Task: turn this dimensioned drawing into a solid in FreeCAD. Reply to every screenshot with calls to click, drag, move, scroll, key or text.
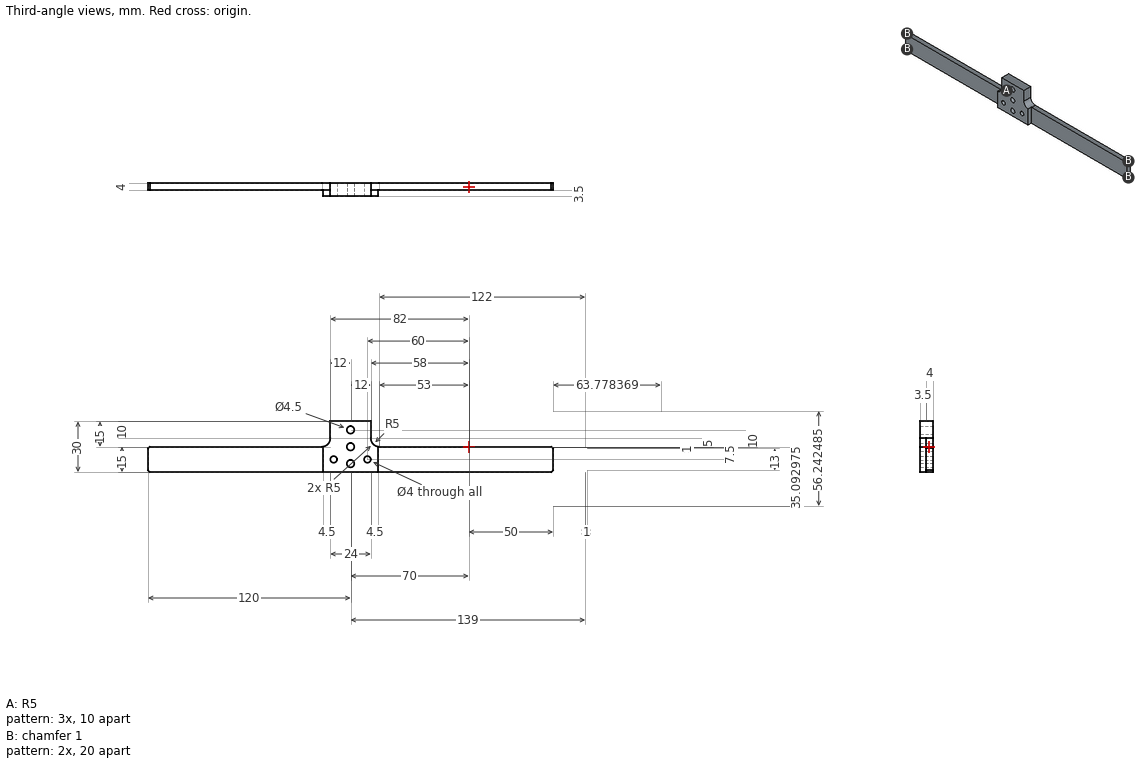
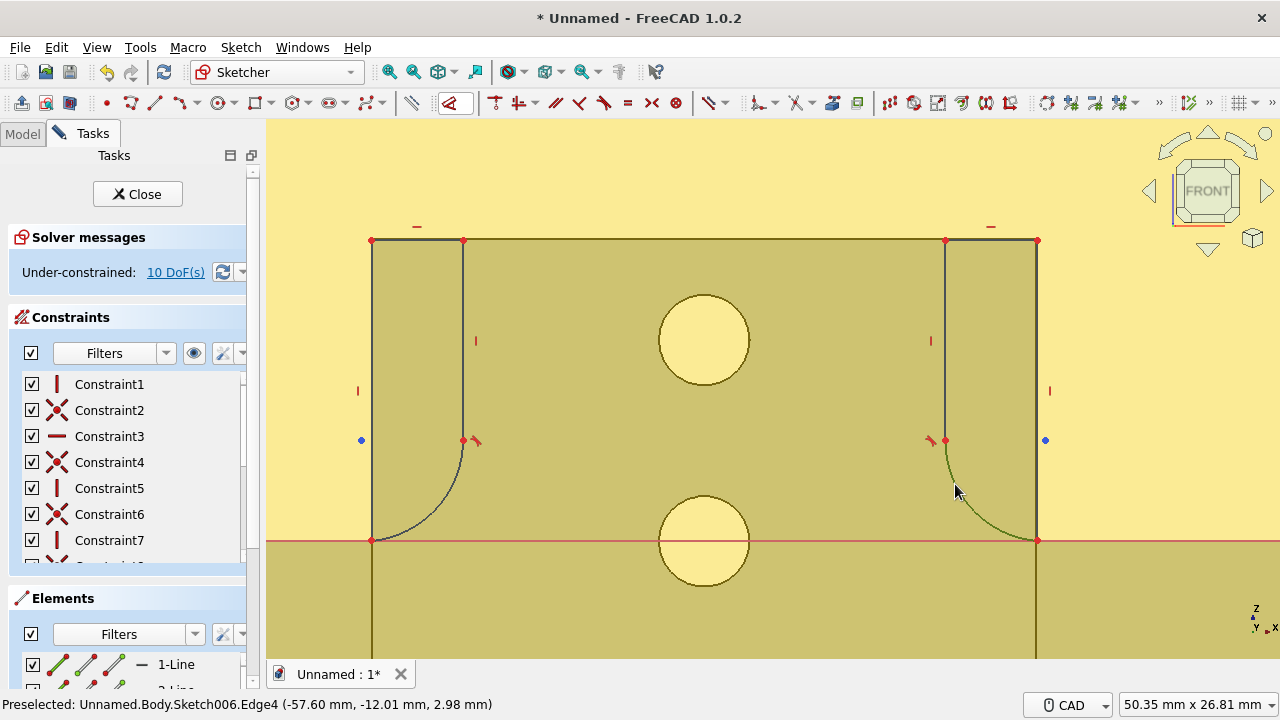
click(414, 527)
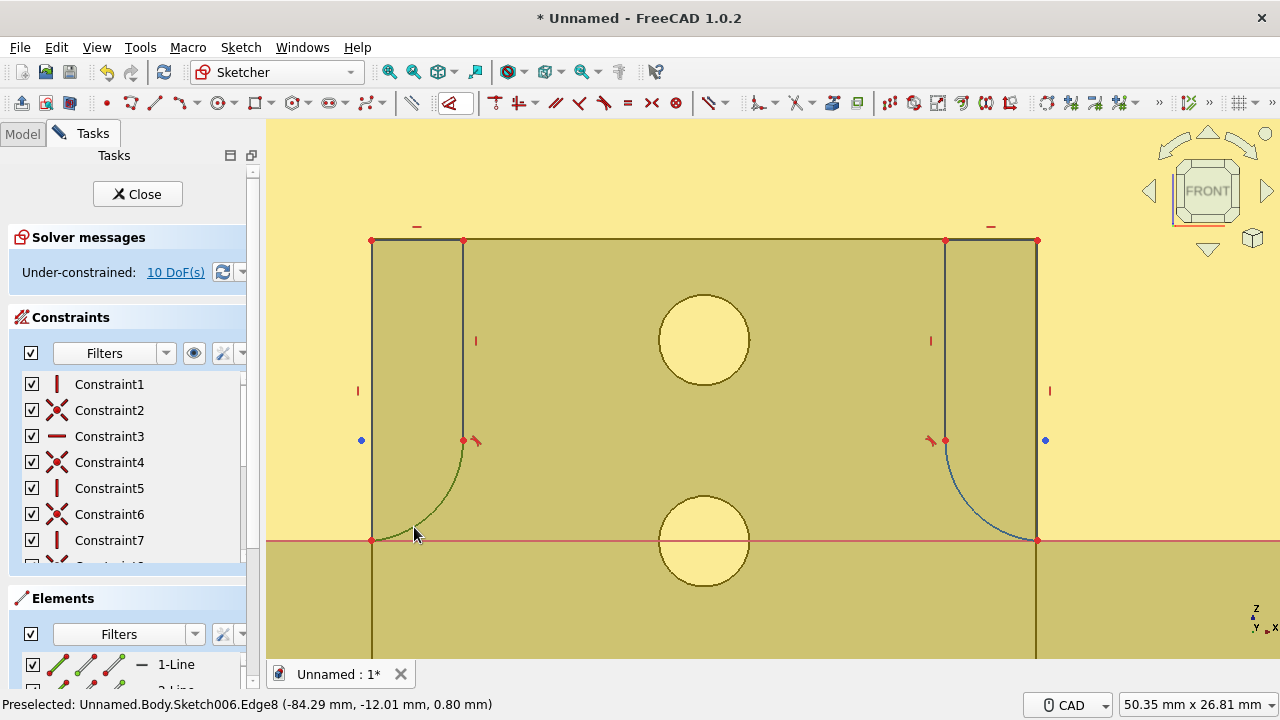
click(628, 104)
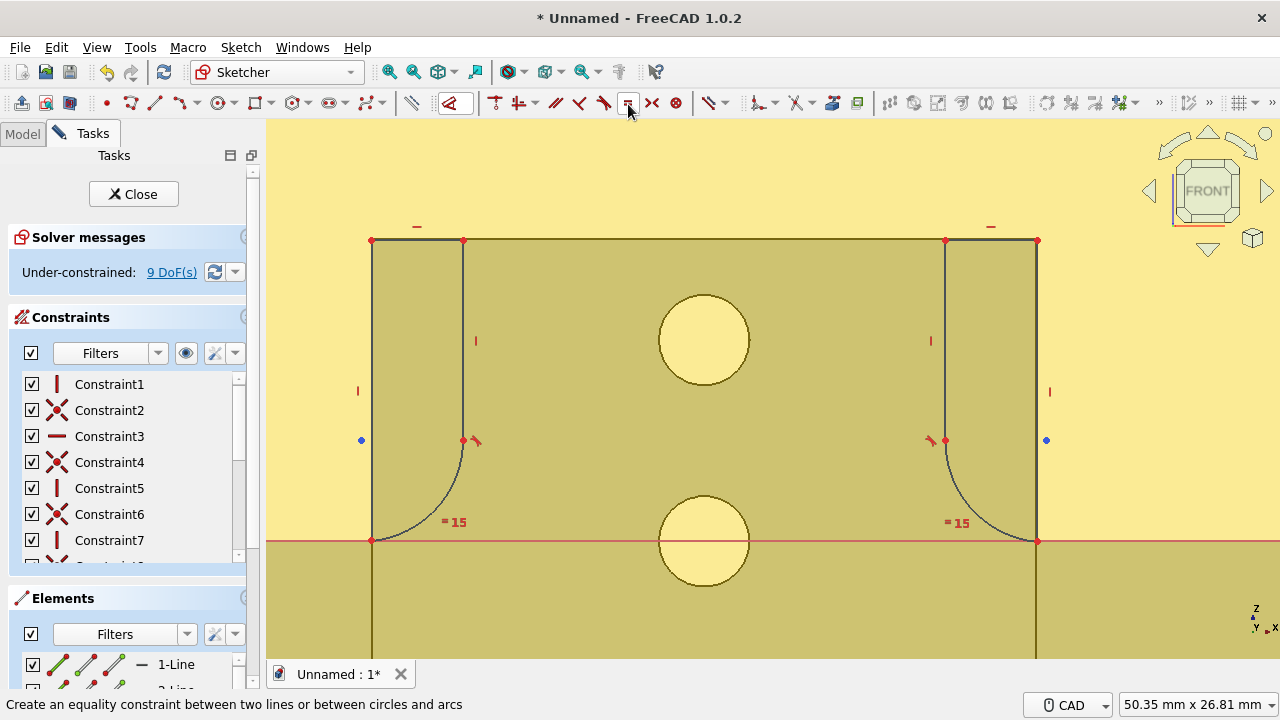
click(955, 484)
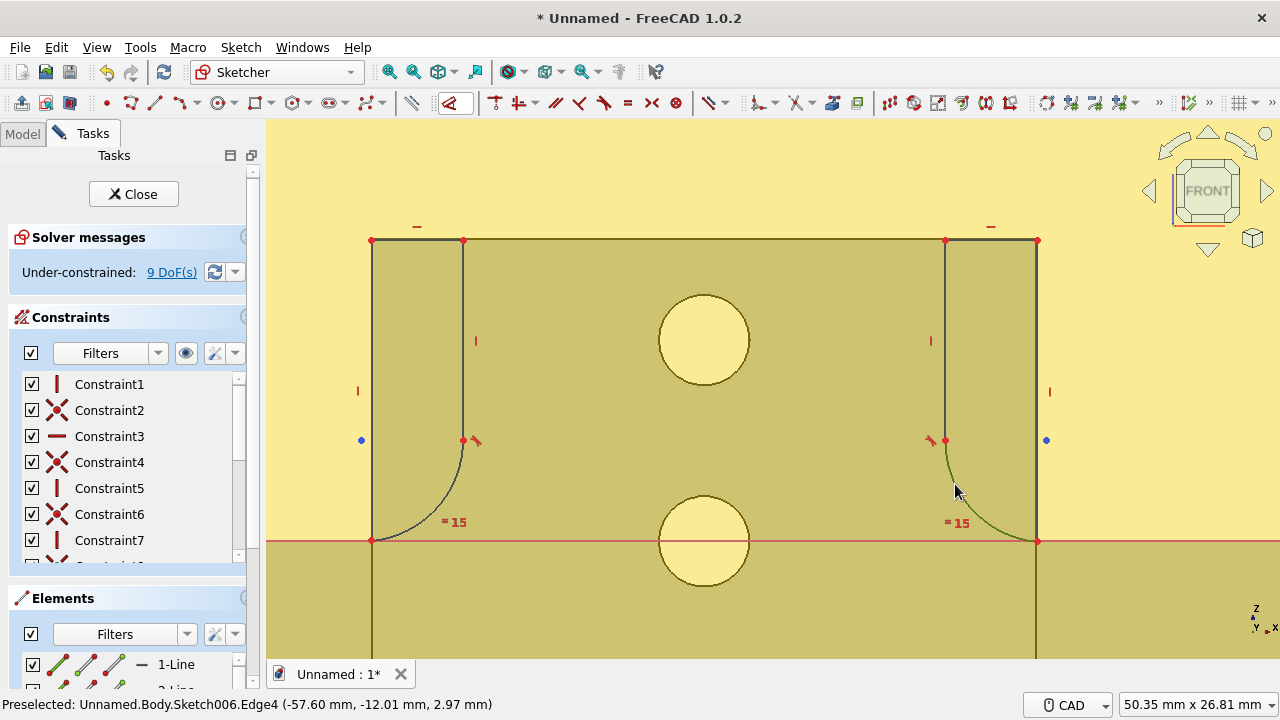
click(468, 104)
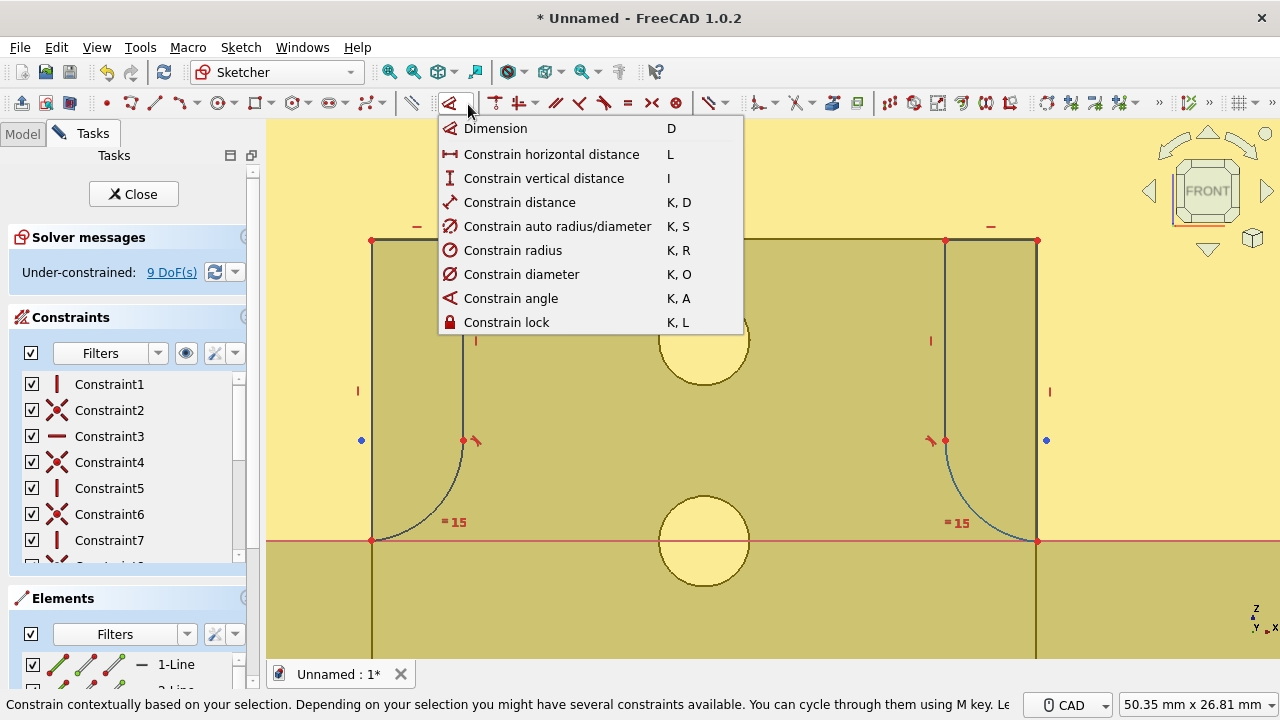
click(591, 250)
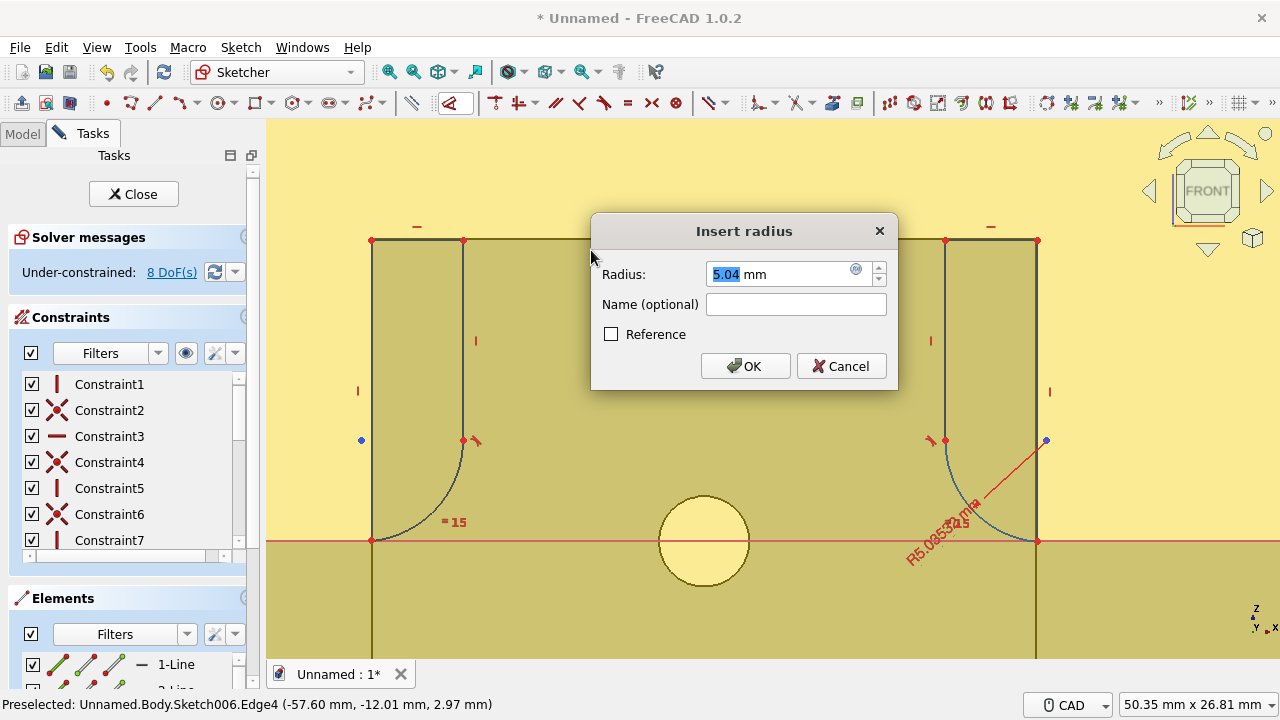
text(5)
key(Return)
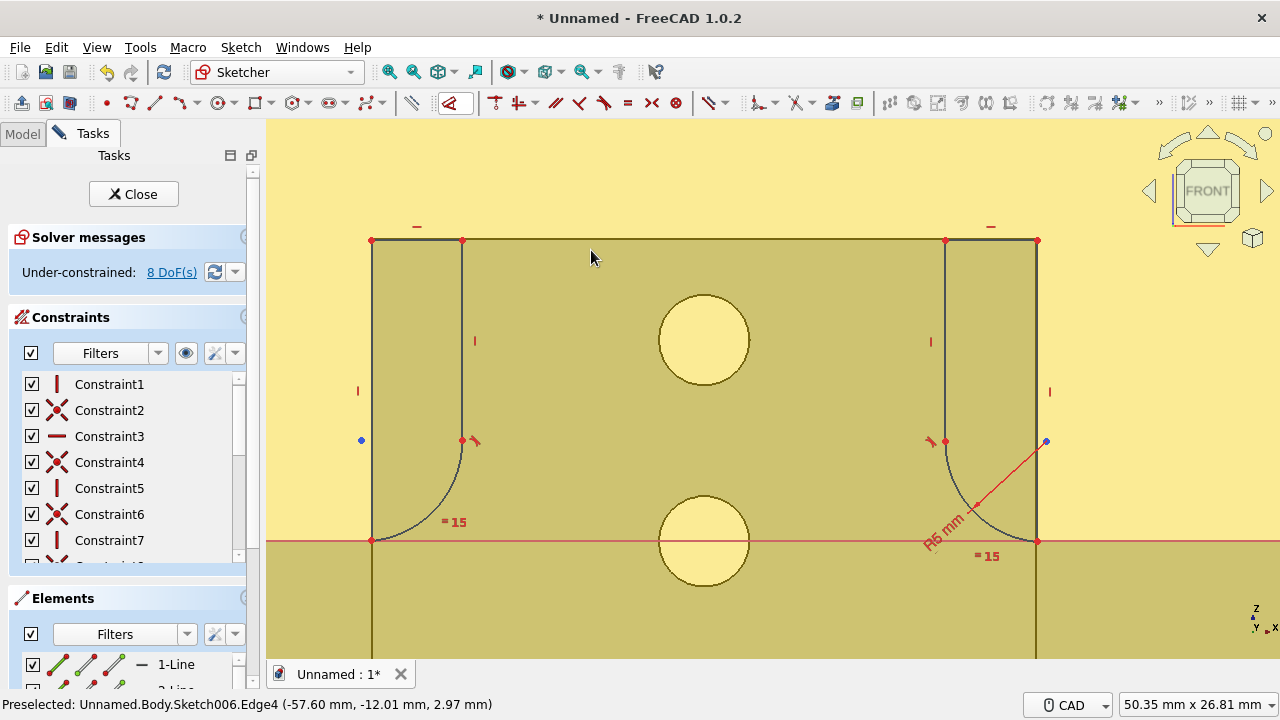
click(945, 381)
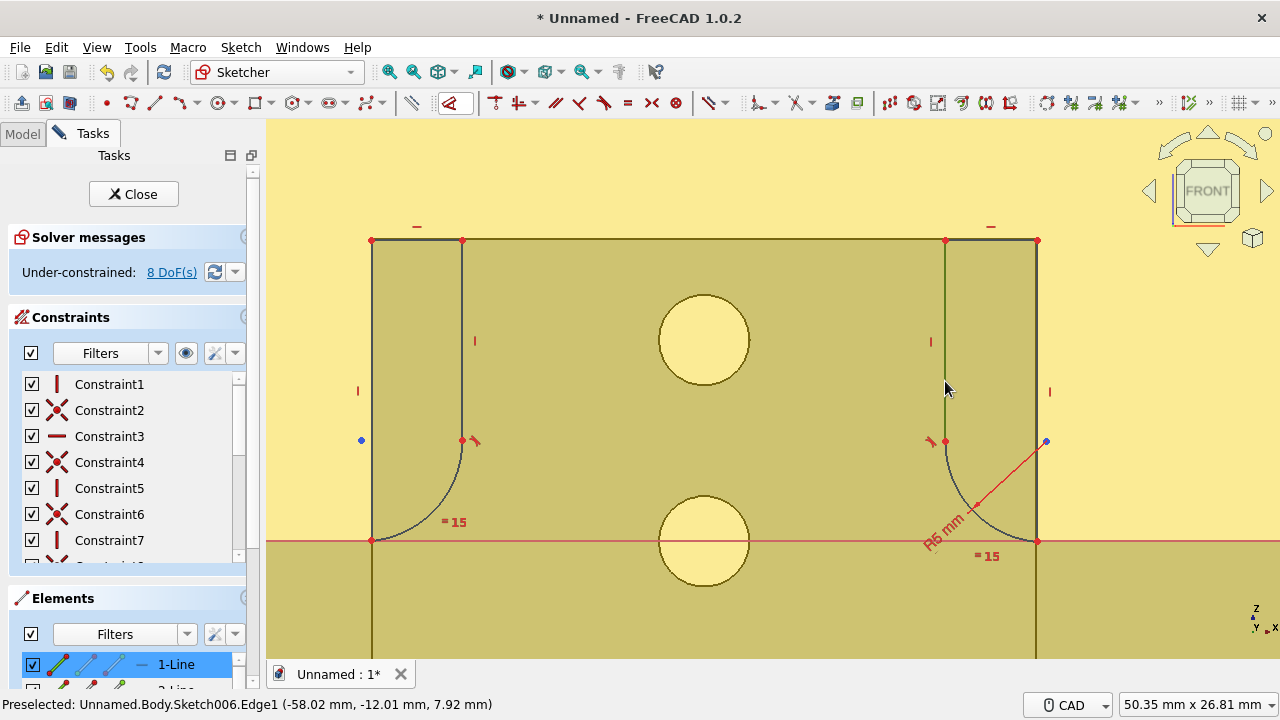
click(468, 104)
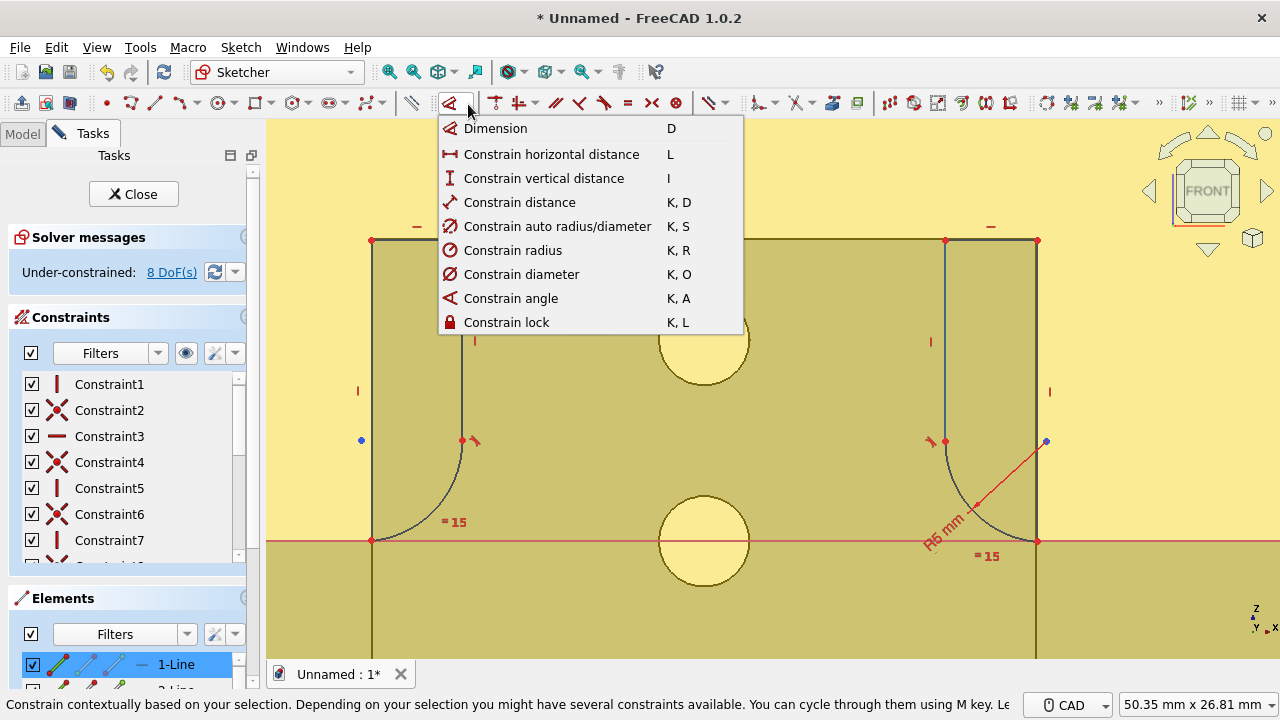
click(591, 178)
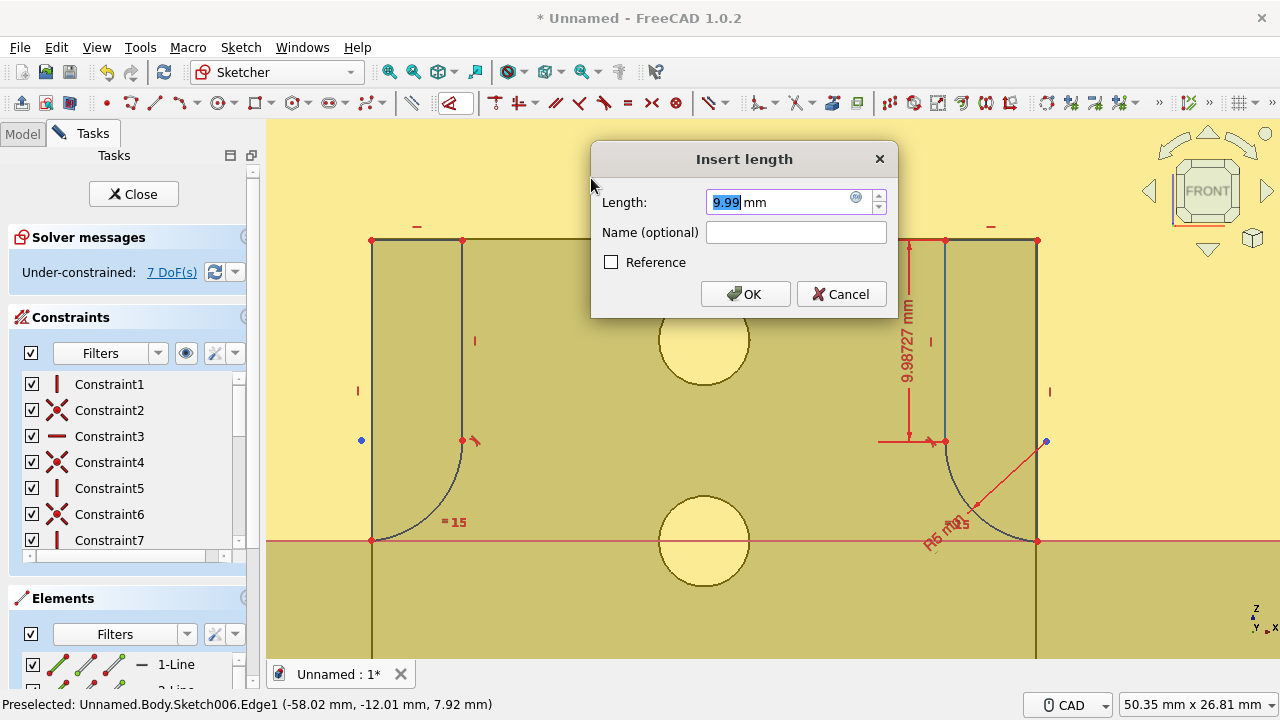
text(10)
key(Return)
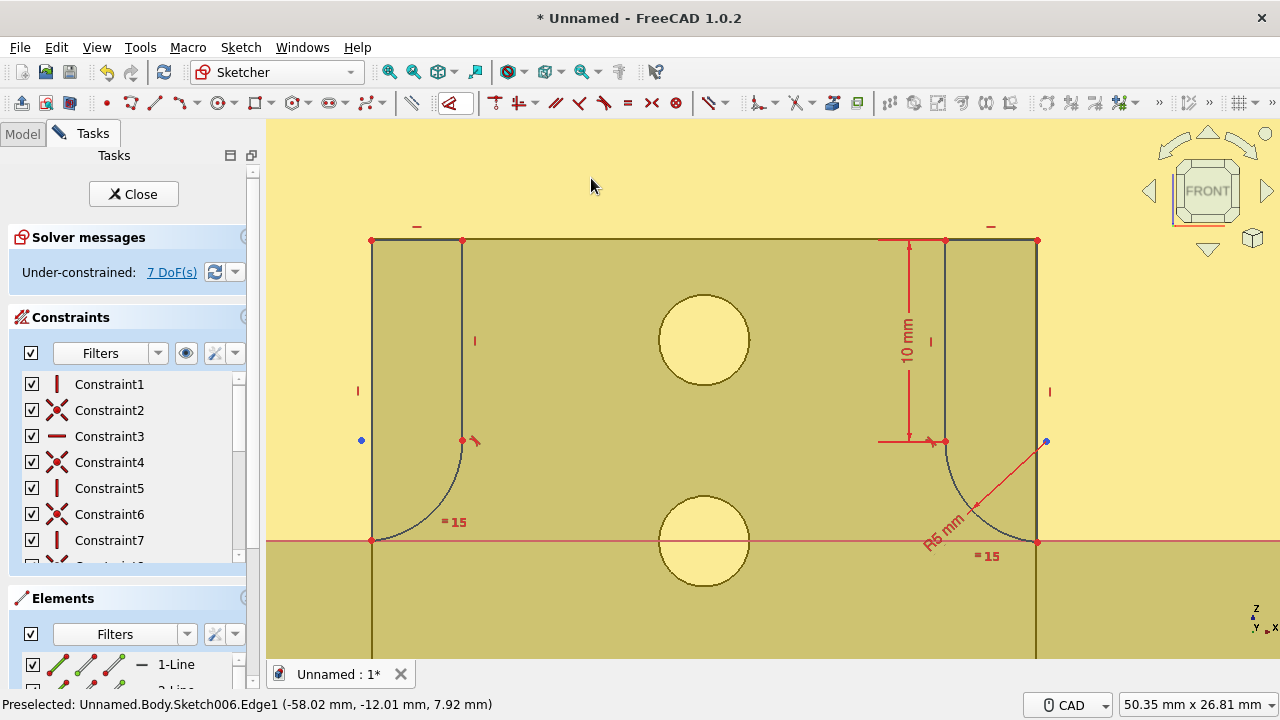
click(462, 300)